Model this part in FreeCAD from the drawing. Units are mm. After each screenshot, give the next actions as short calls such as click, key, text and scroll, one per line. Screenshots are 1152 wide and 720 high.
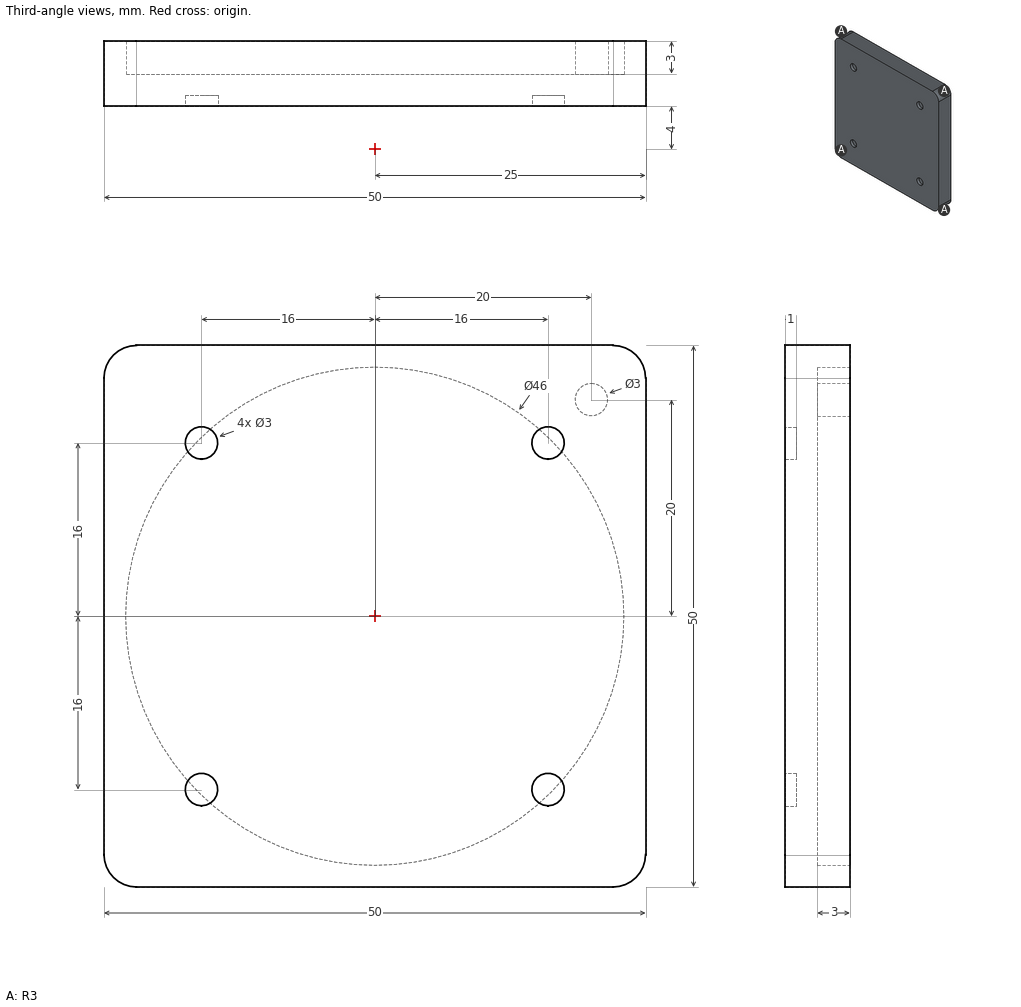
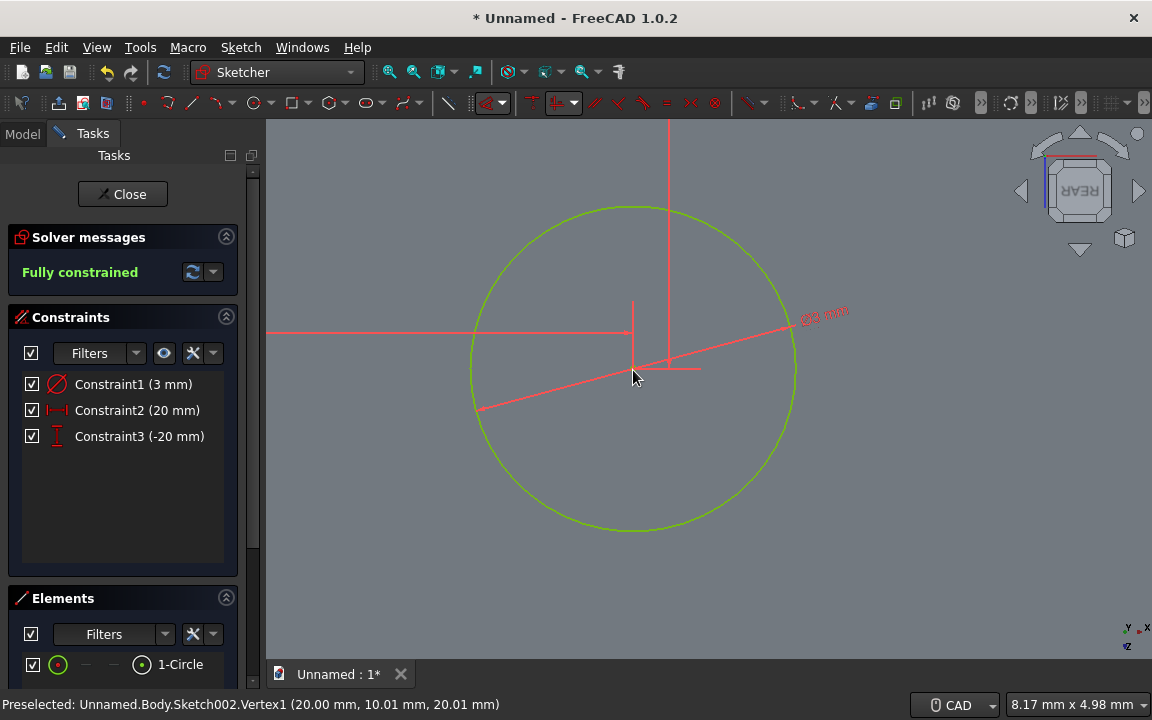
click(123, 194)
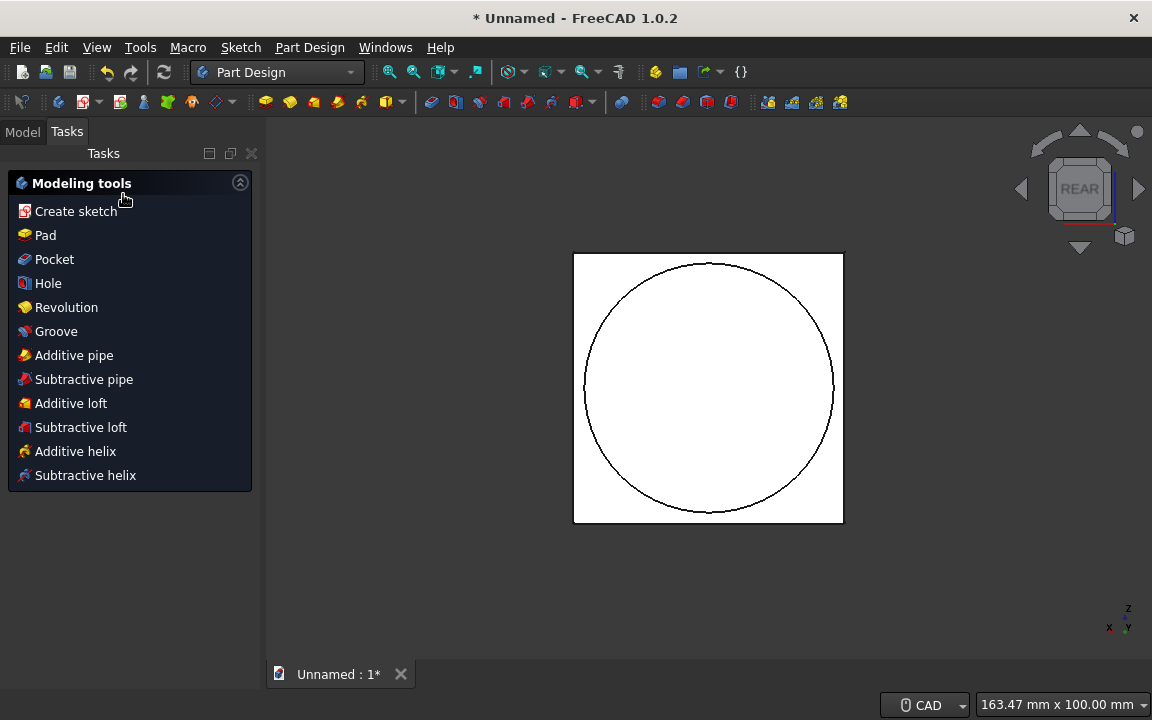
click(432, 102)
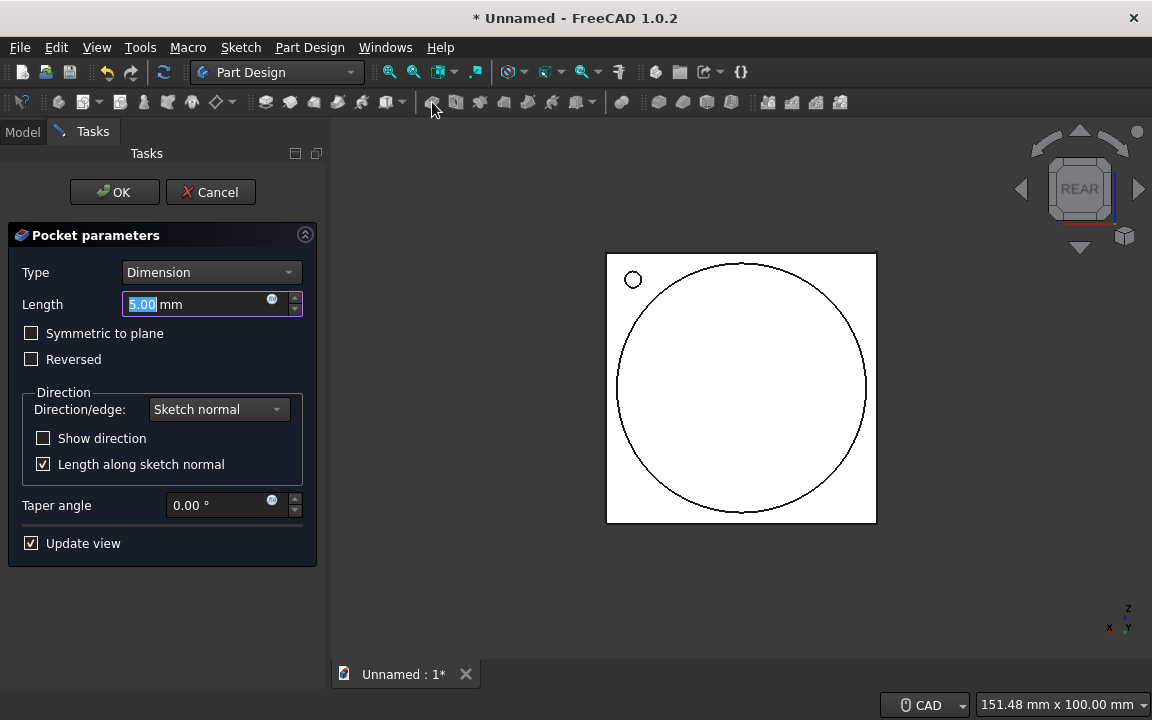
text(3)
key(Tab)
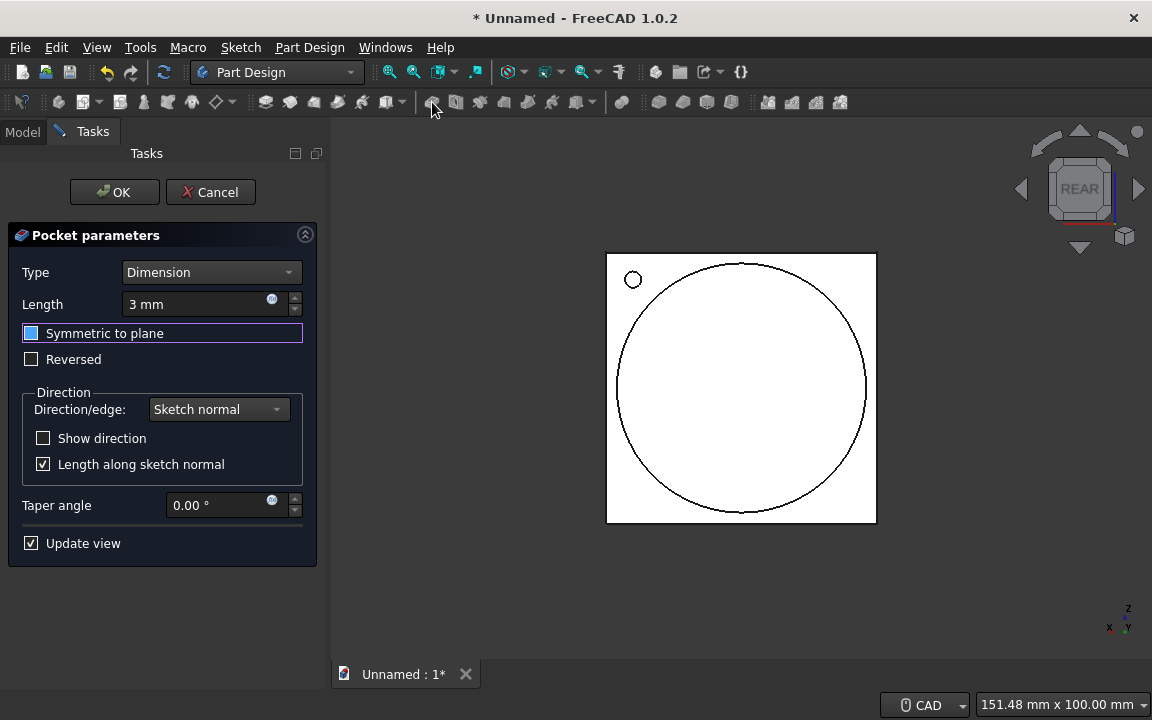
click(115, 192)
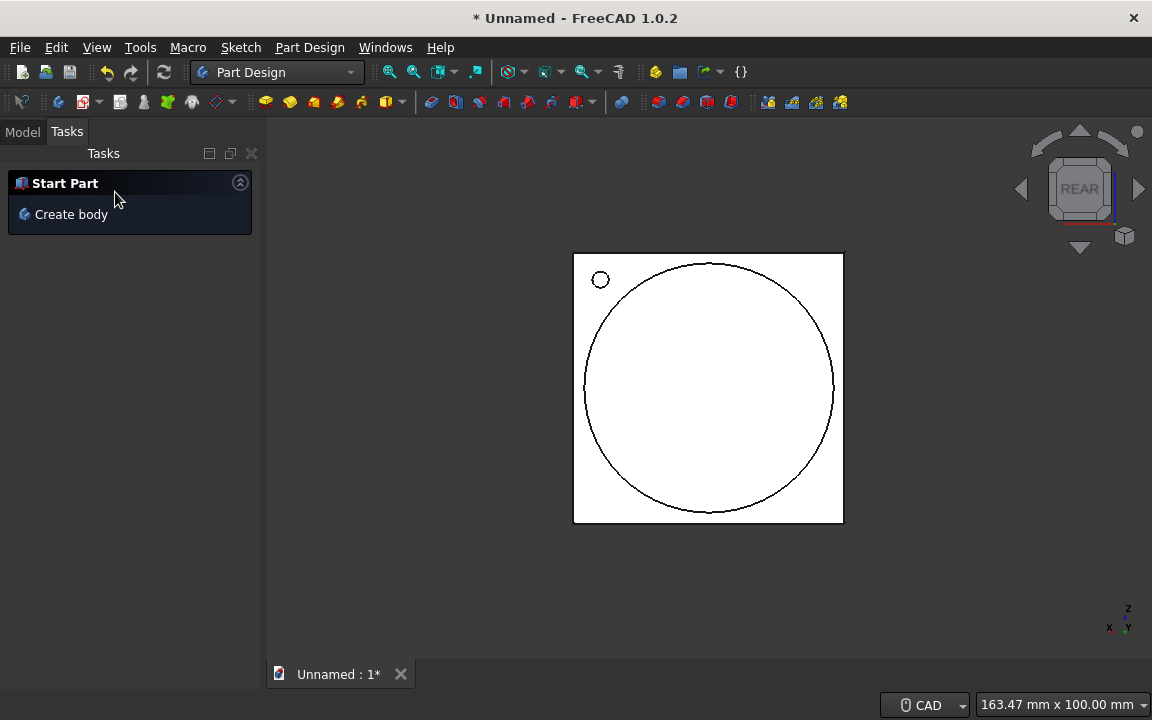
key(0)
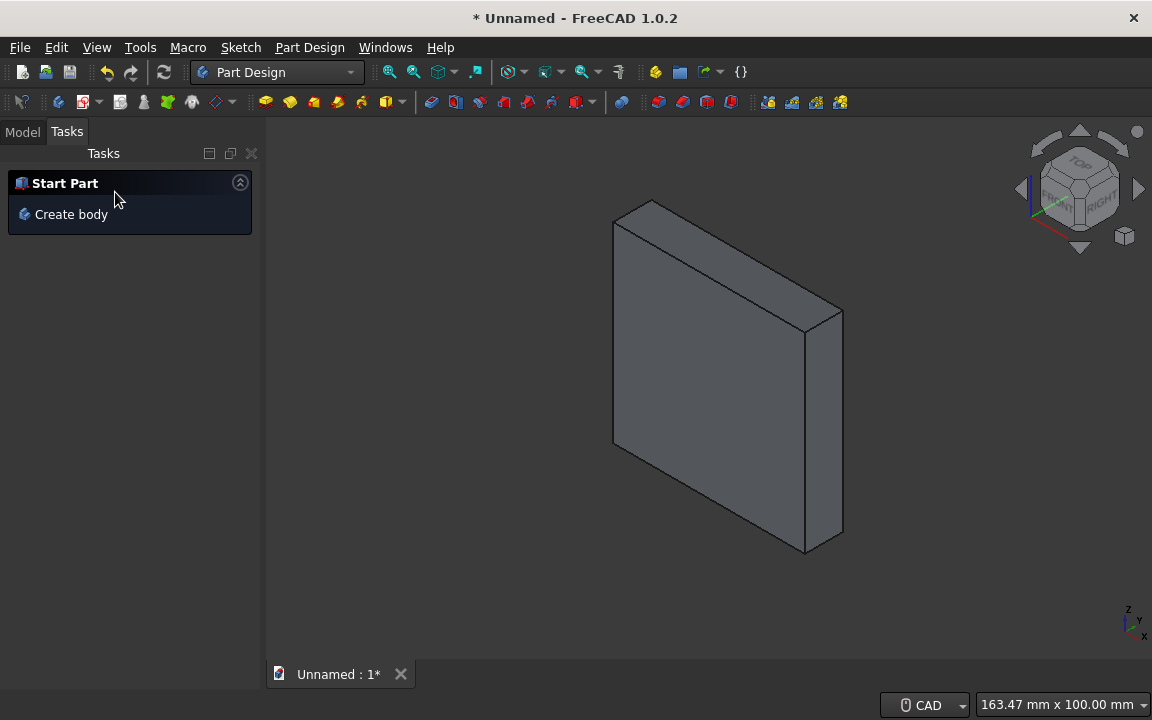
click(783, 297)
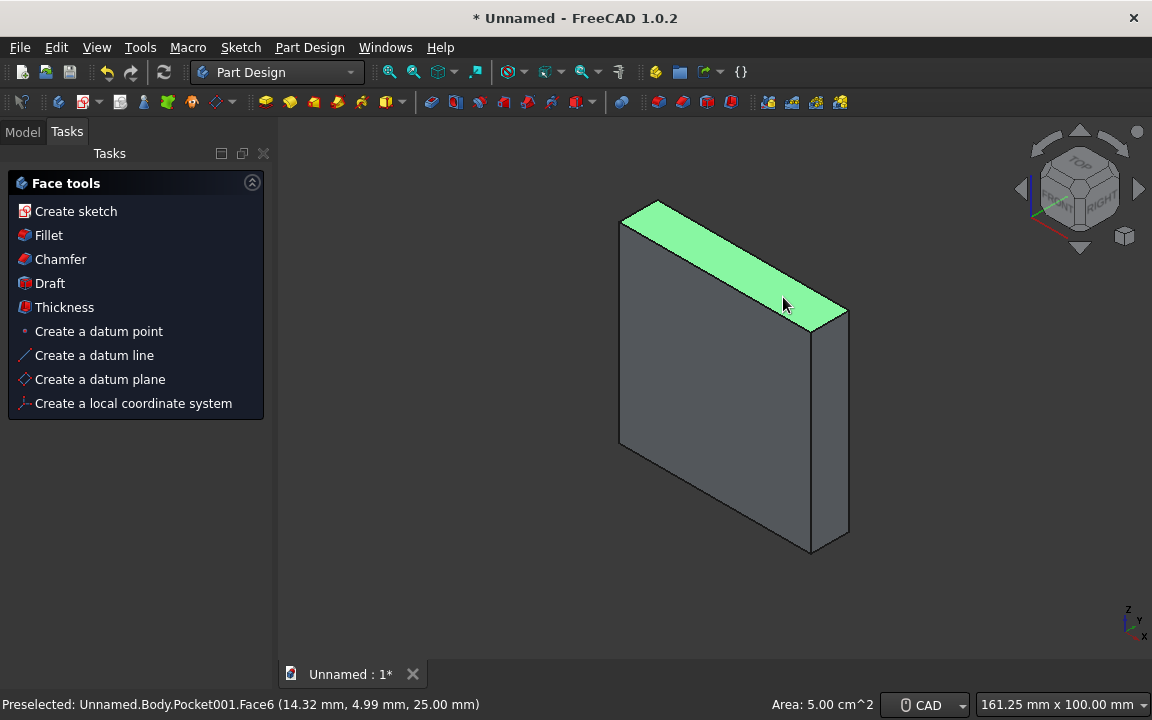
click(84, 102)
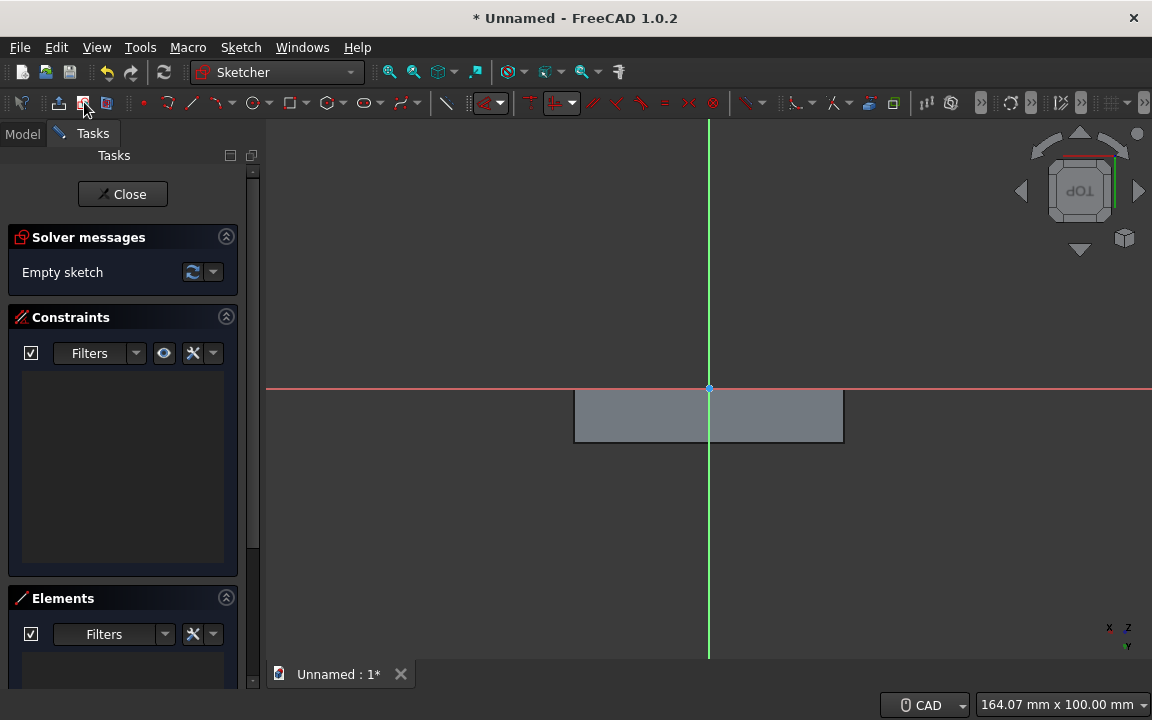
scroll(792, 413, up, 3)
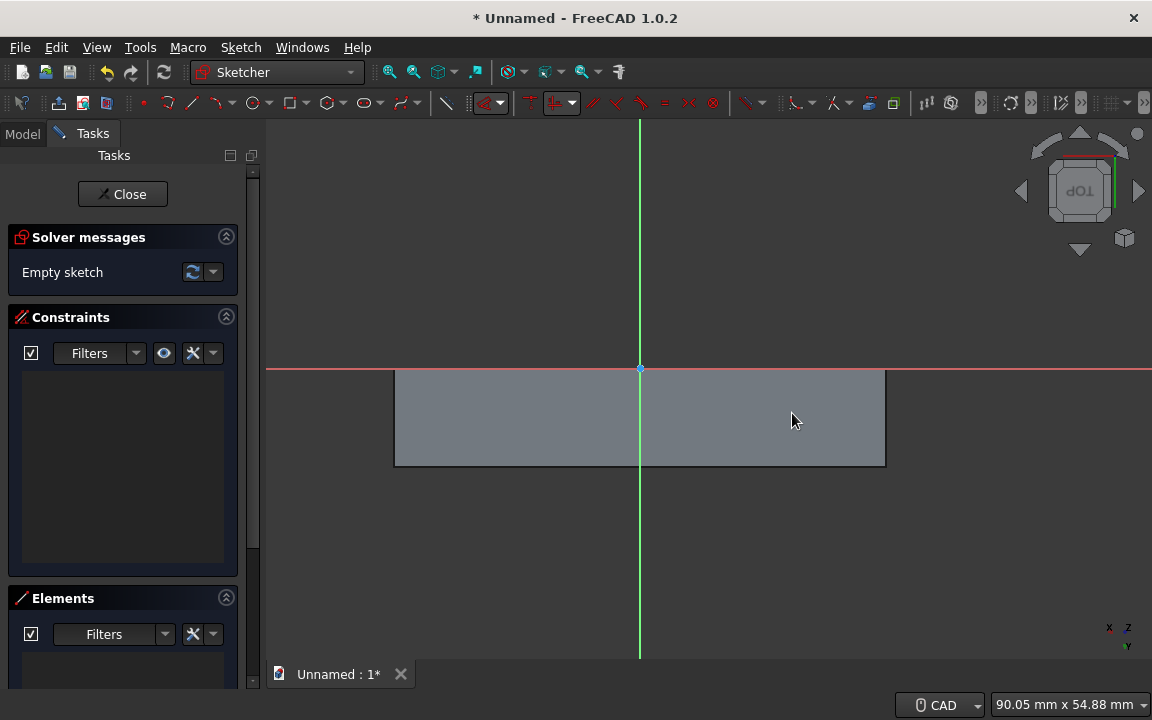
click(290, 104)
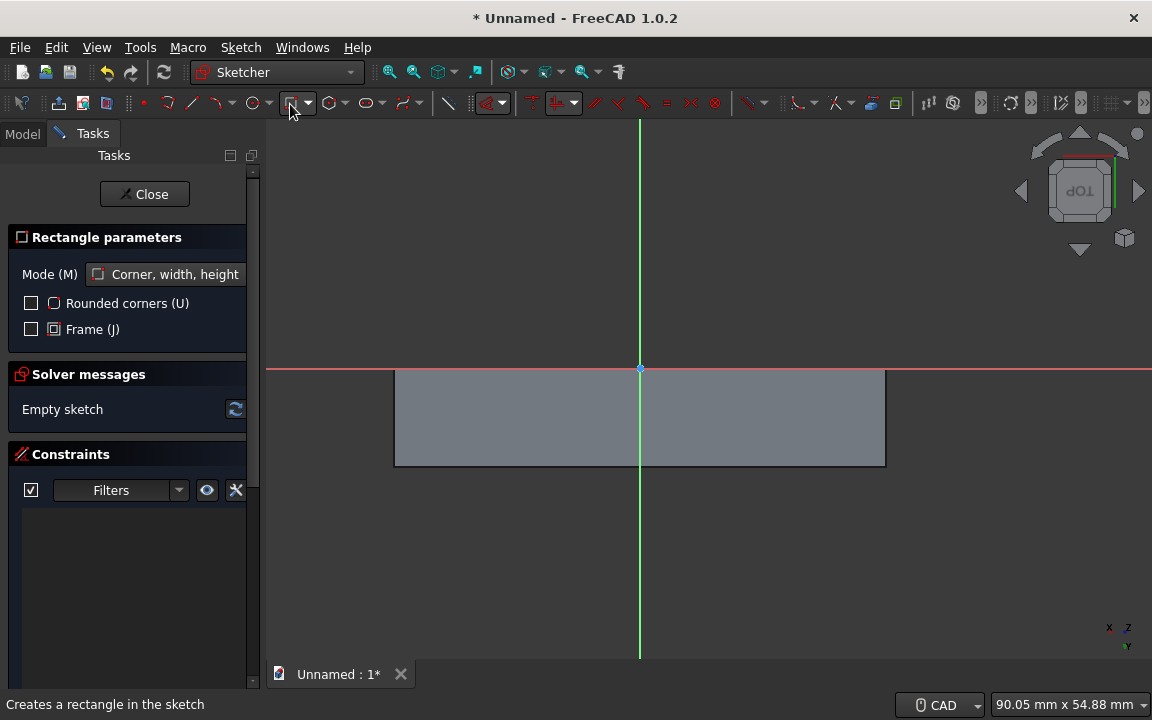
click(394, 369)
click(886, 408)
key(Escape)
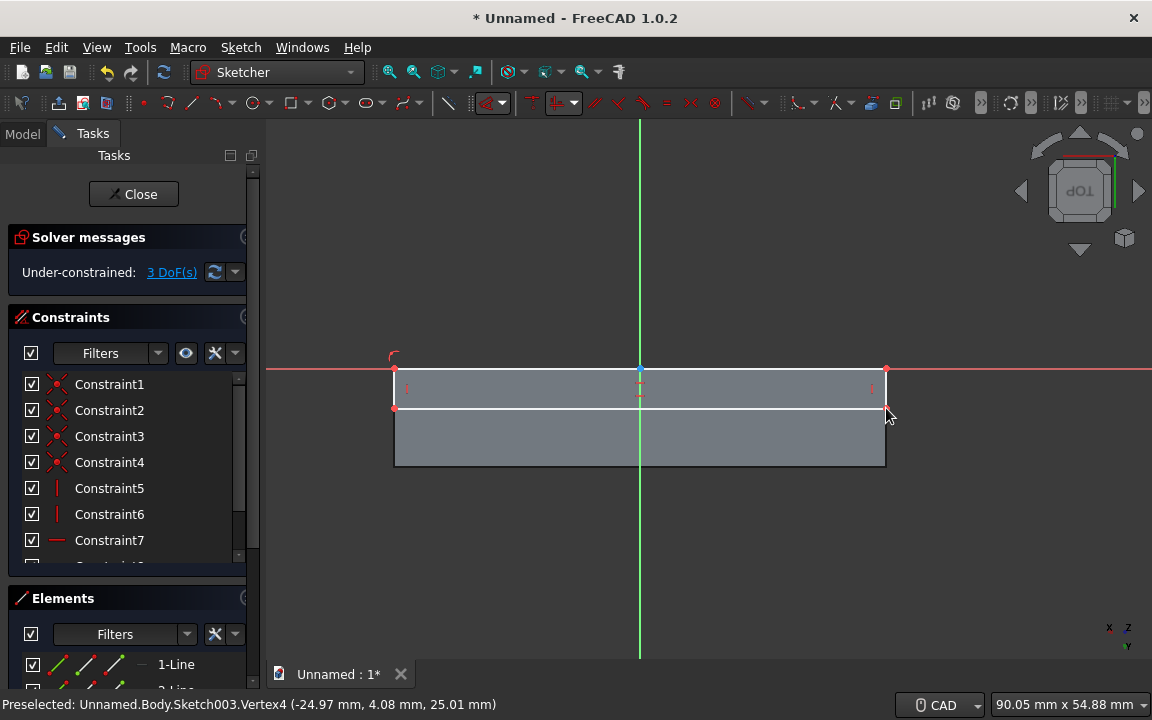
click(394, 381)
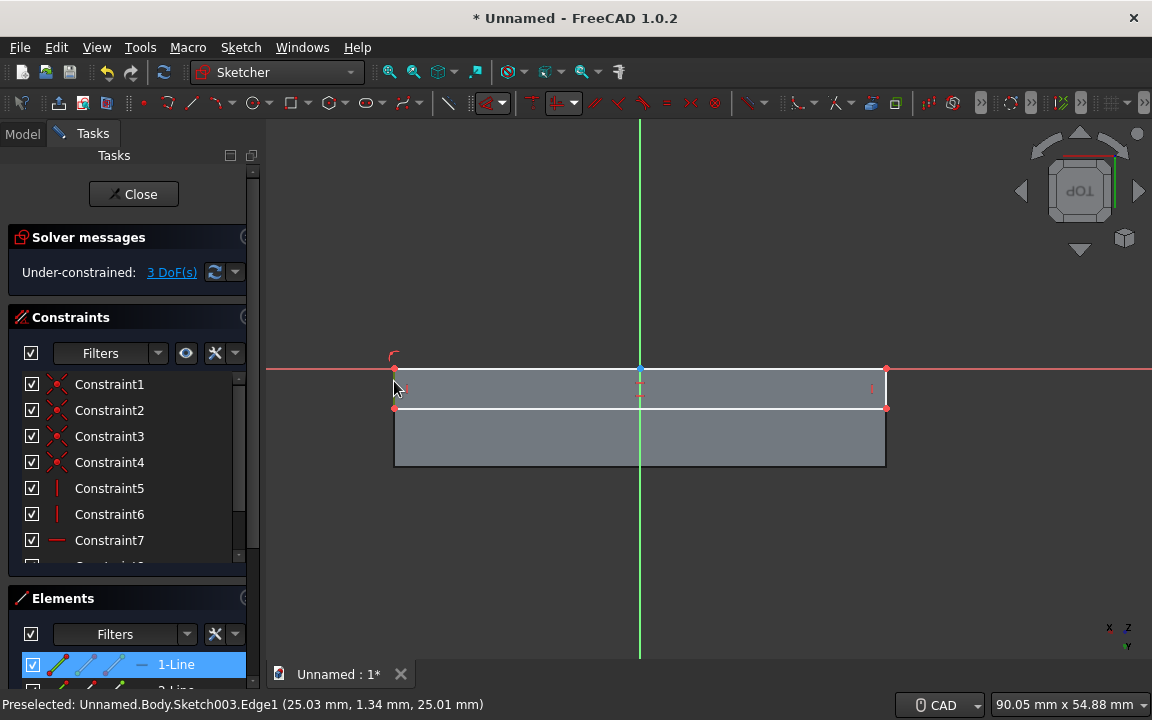
click(504, 104)